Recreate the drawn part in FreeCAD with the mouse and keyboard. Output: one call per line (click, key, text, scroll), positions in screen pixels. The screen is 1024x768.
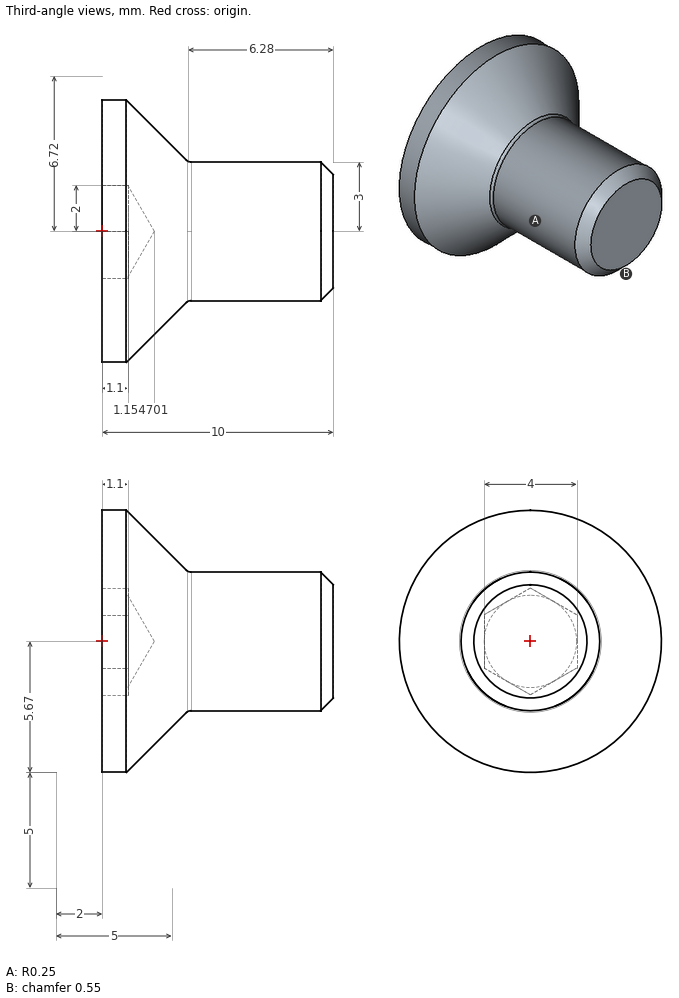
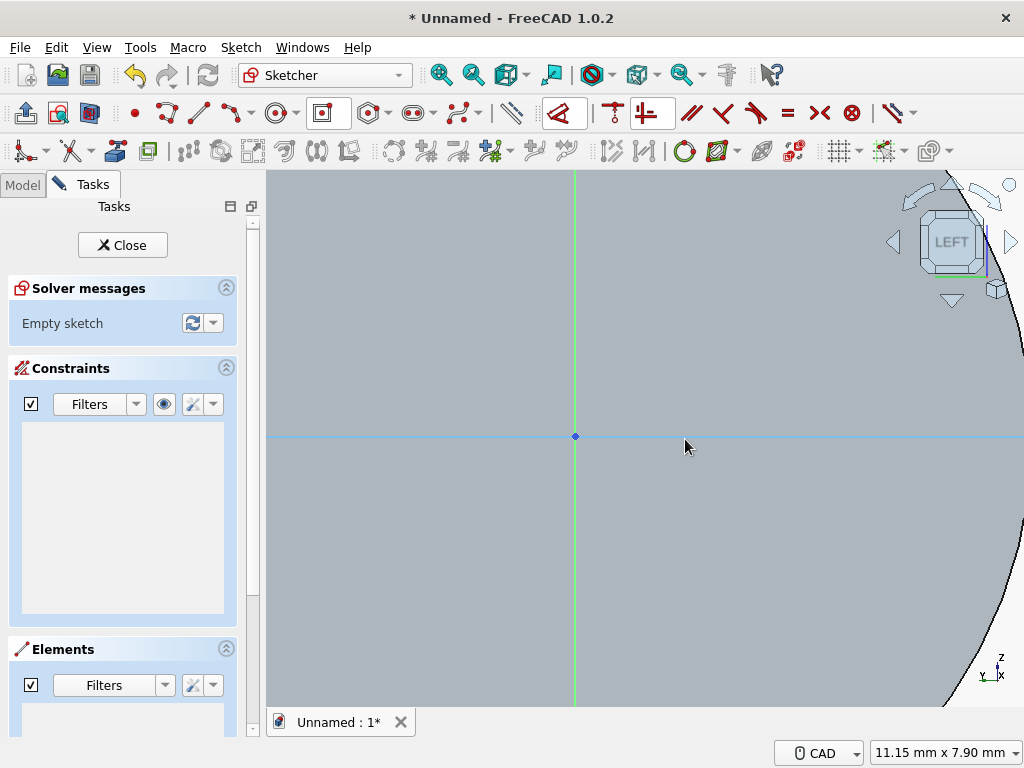
click(368, 114)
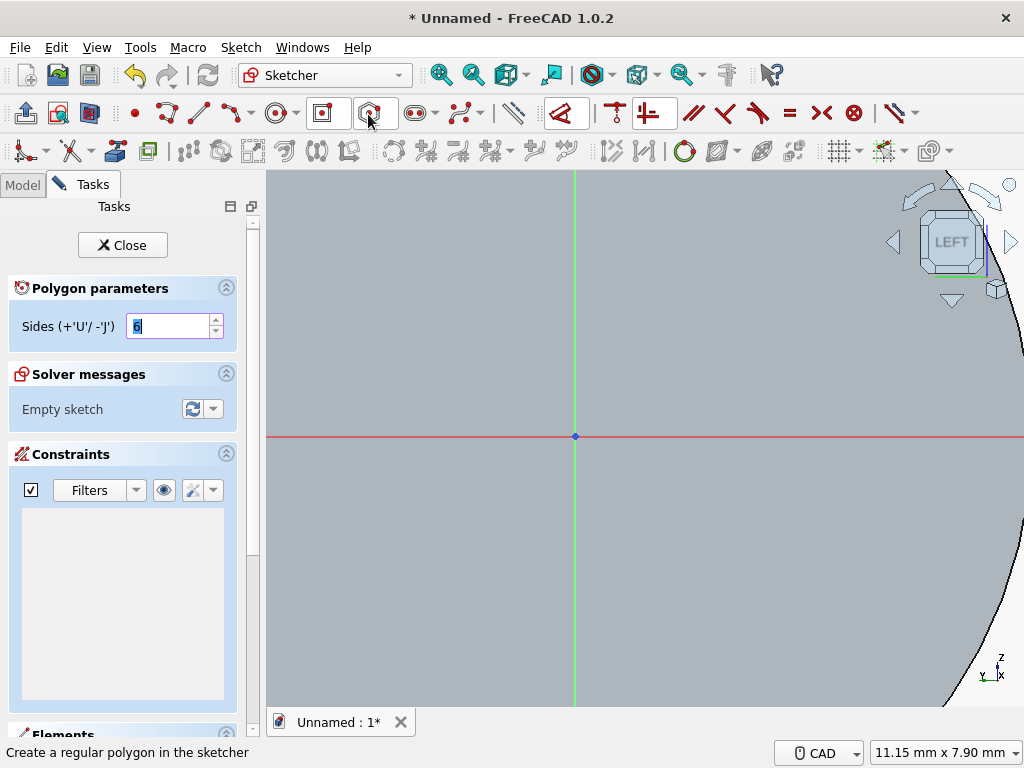
click(575, 437)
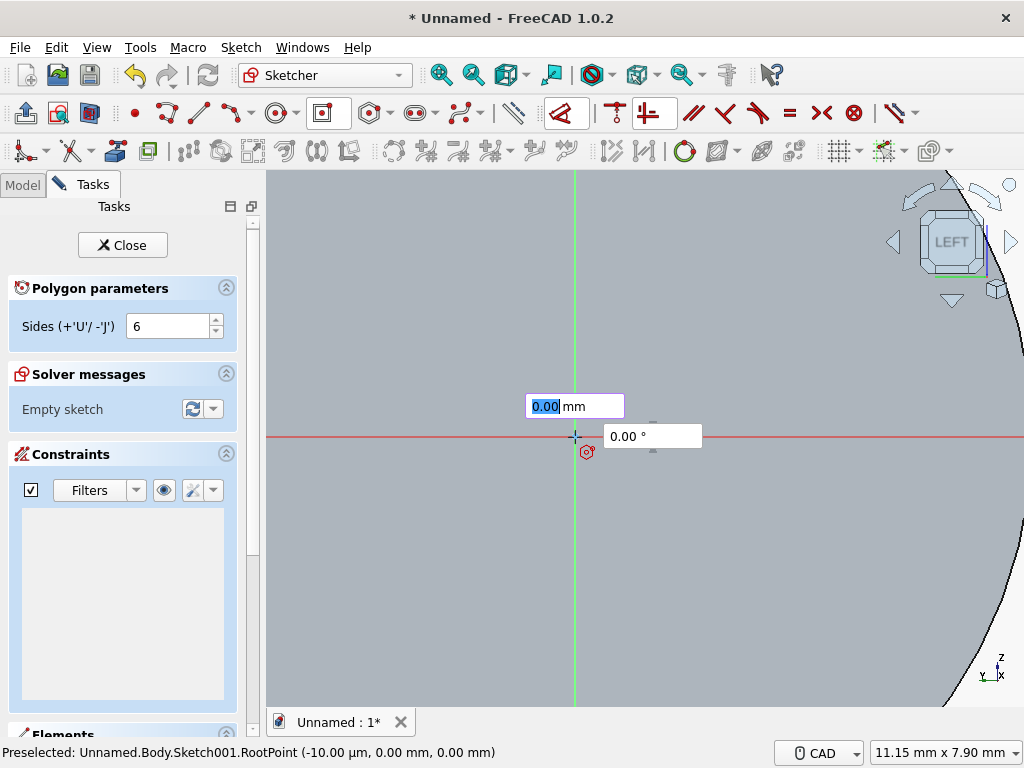
click(575, 594)
key(Escape)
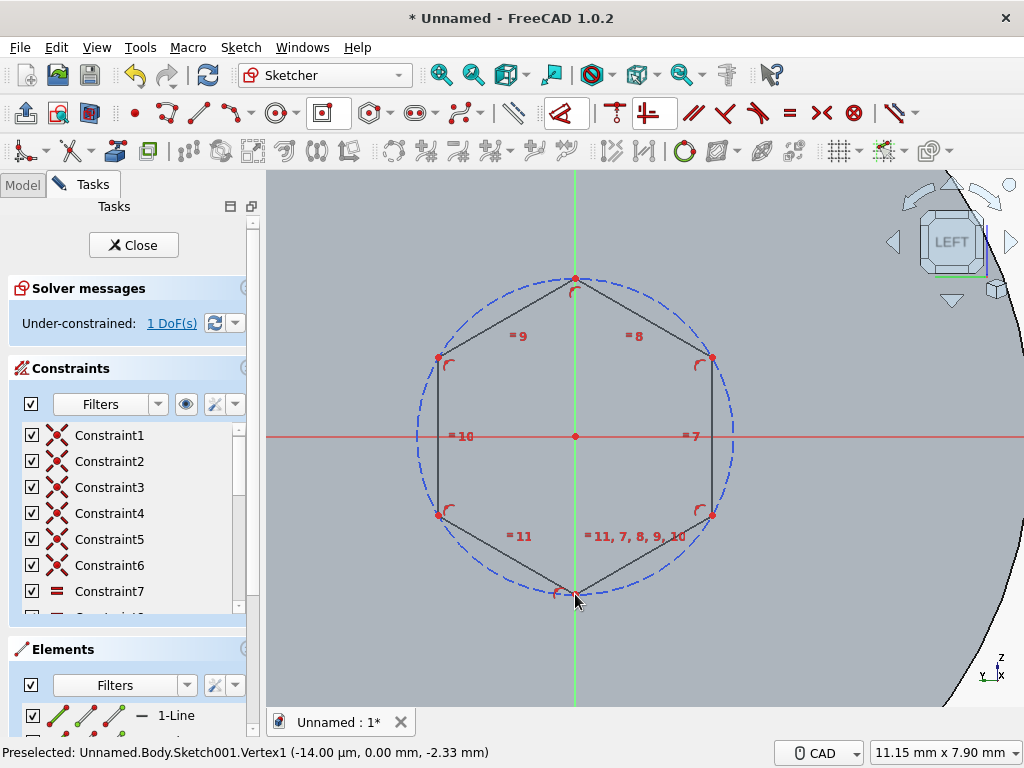
key(d)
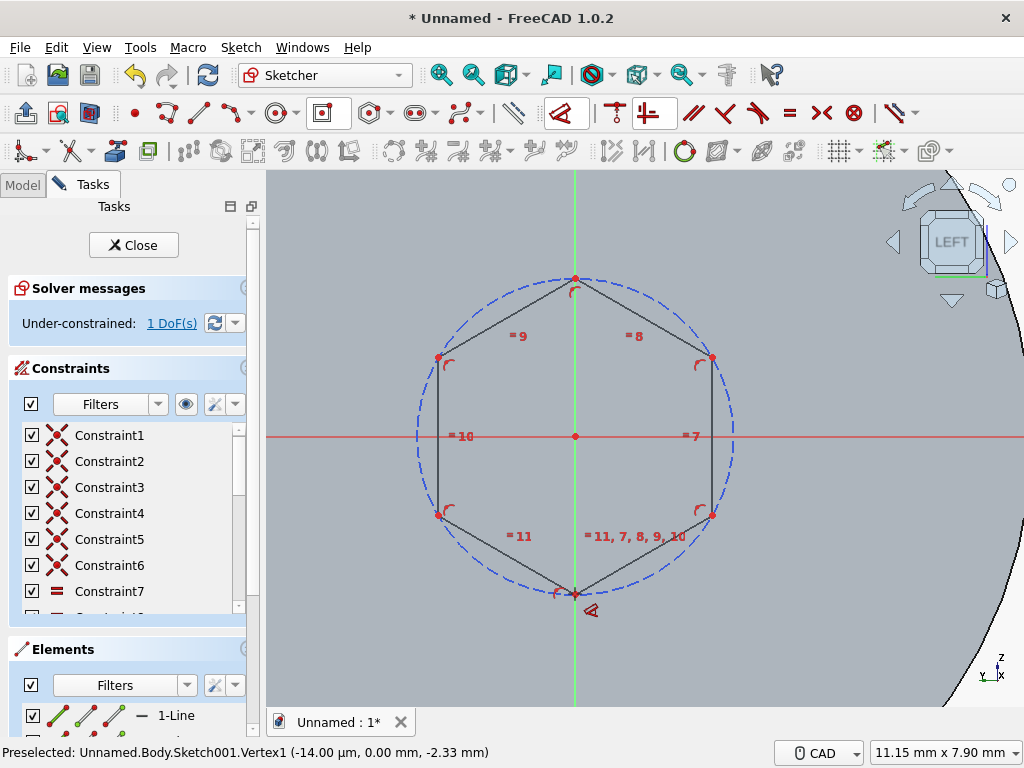
click(438, 358)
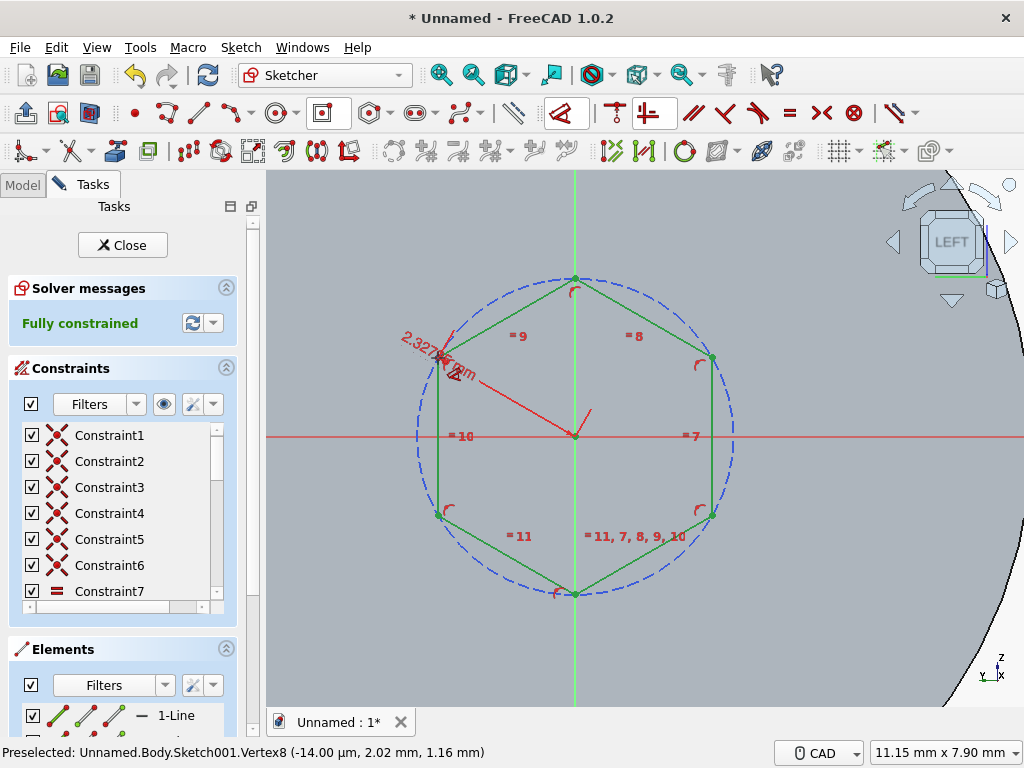
click(712, 516)
click(512, 598)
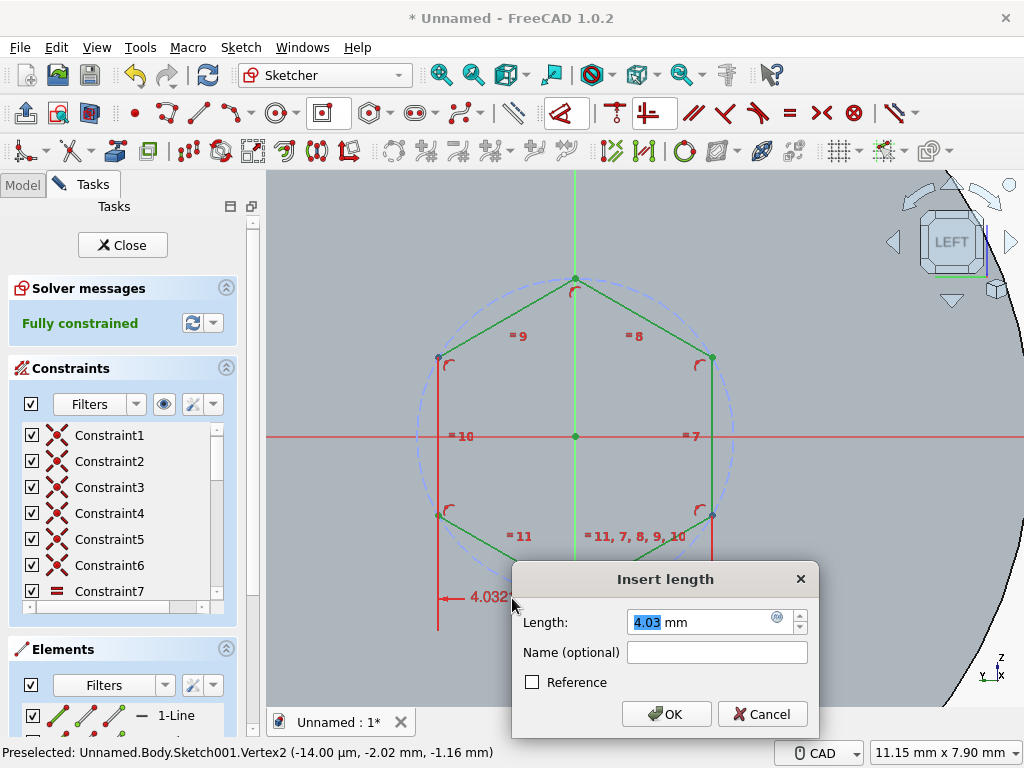
text(4)
key(Return)
key(Escape)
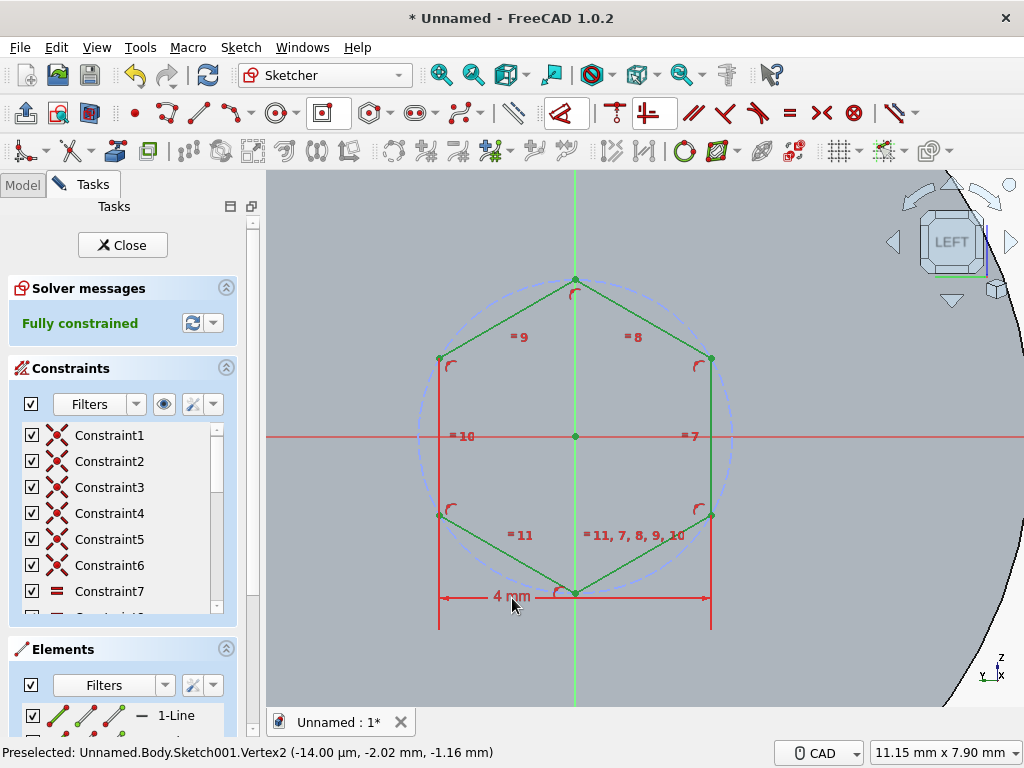
click(123, 245)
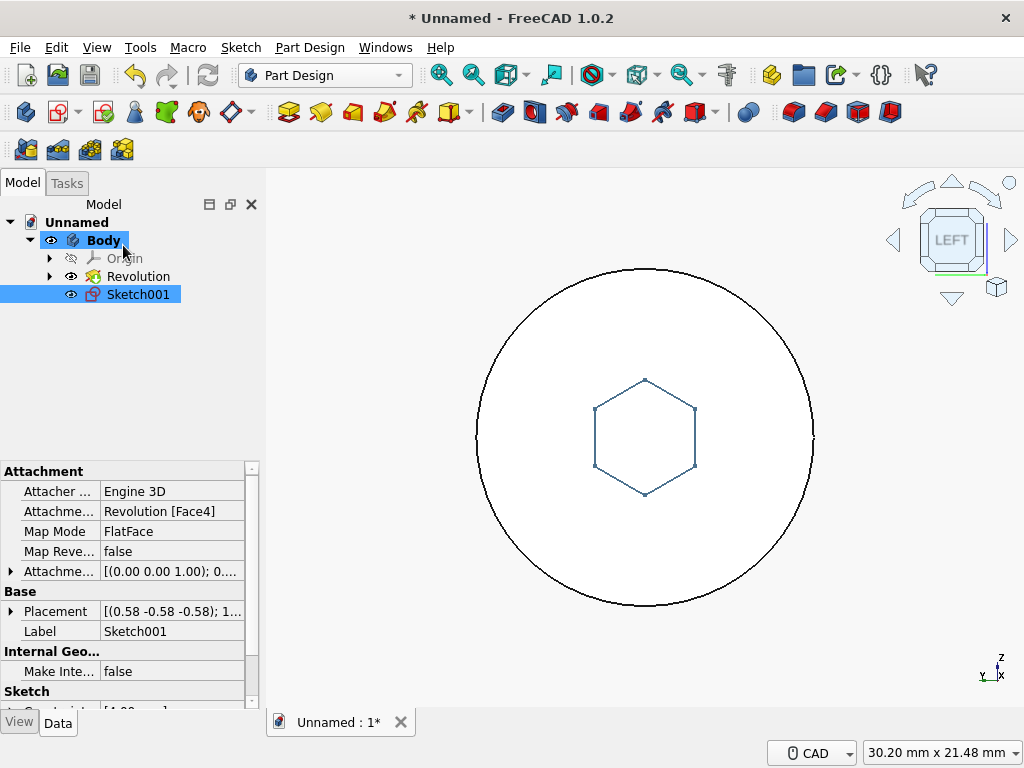
click(504, 112)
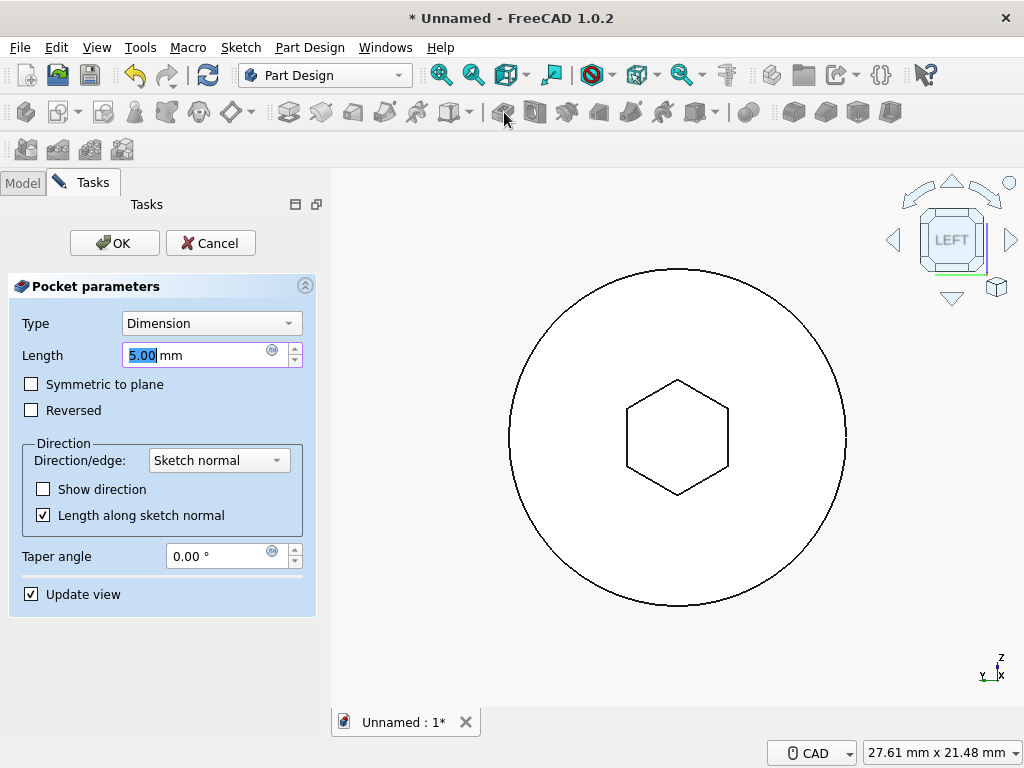
text(1.1)
key(Tab)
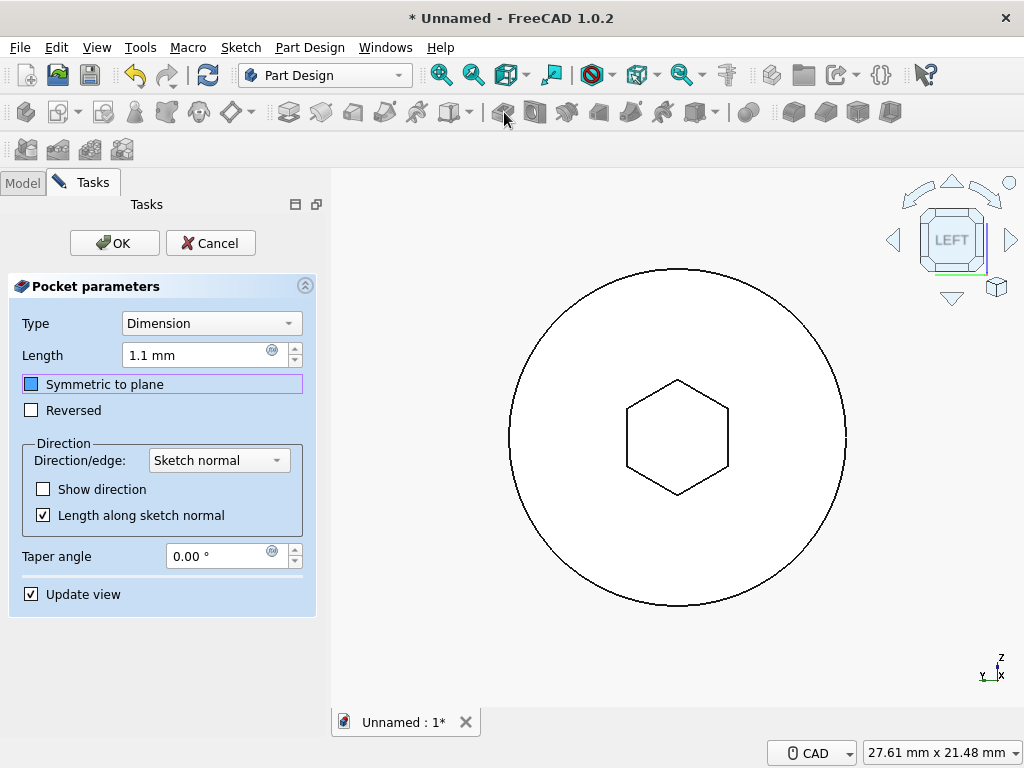
click(115, 243)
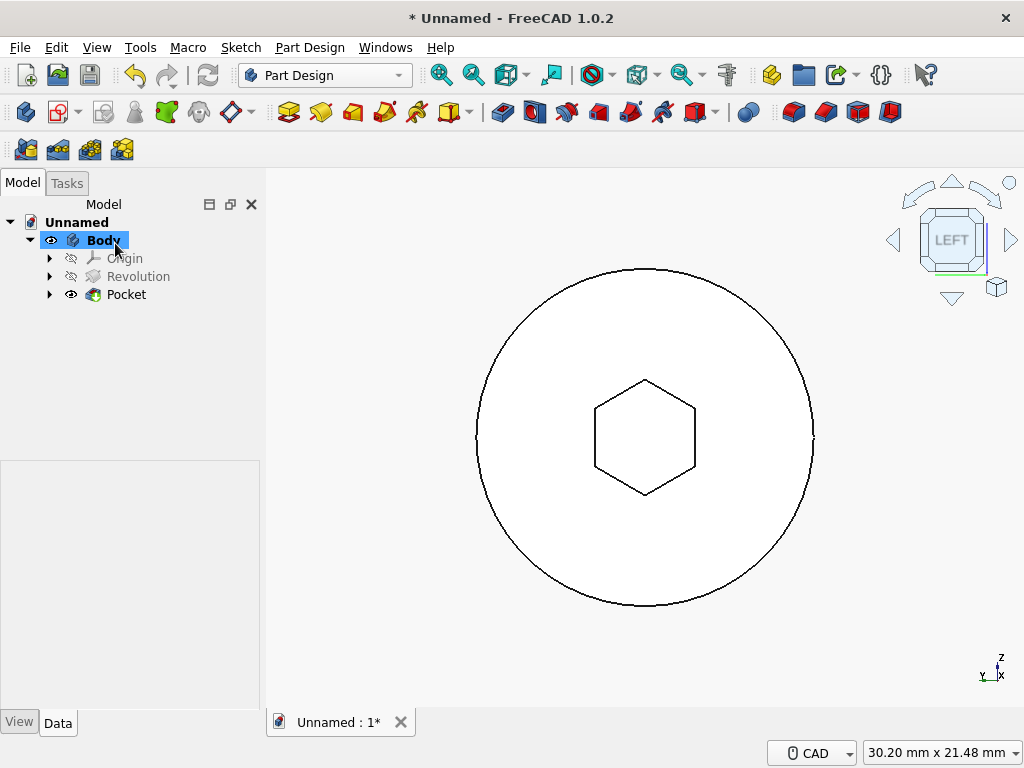
click(58, 112)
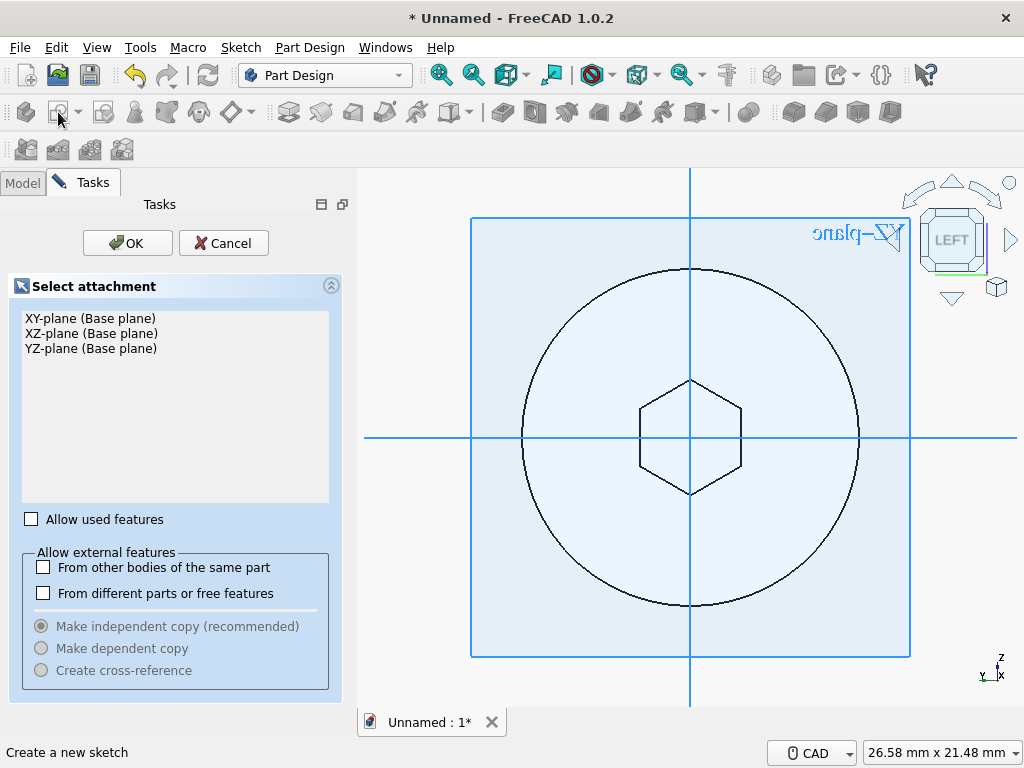
click(82, 318)